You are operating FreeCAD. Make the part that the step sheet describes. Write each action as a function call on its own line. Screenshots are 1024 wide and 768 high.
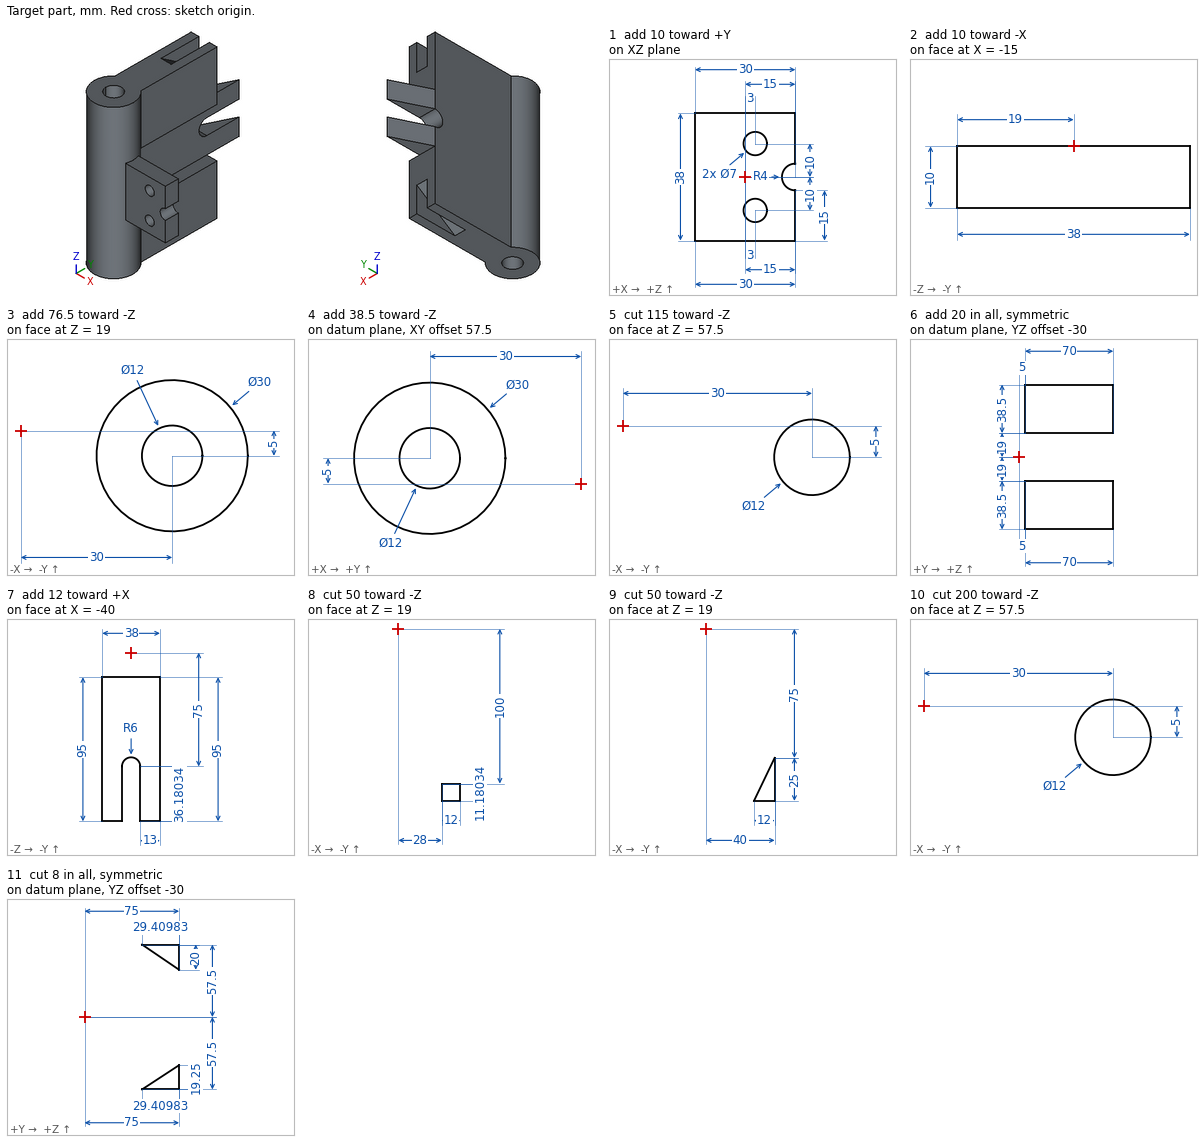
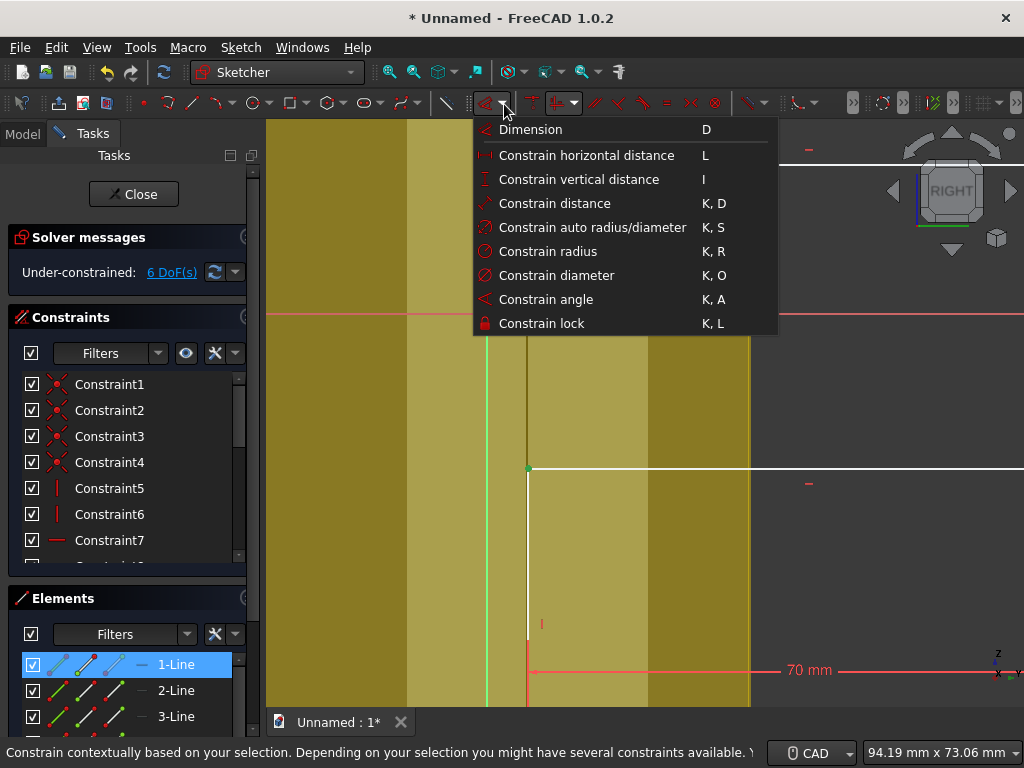
click(626, 155)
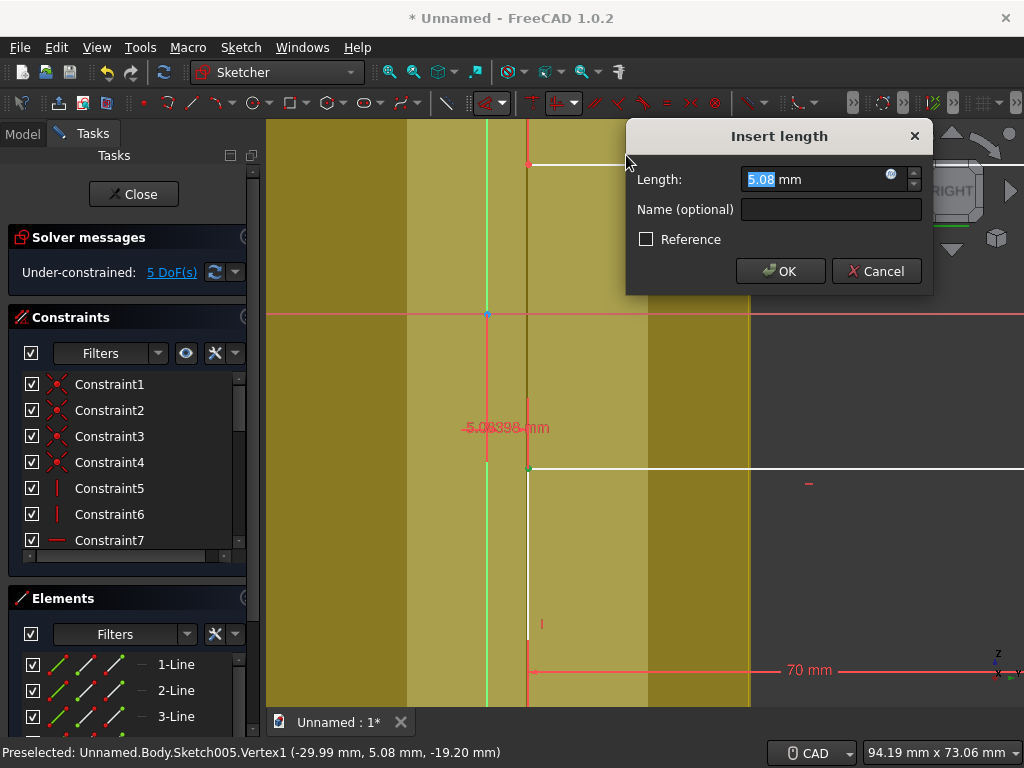
text(5)
key(Return)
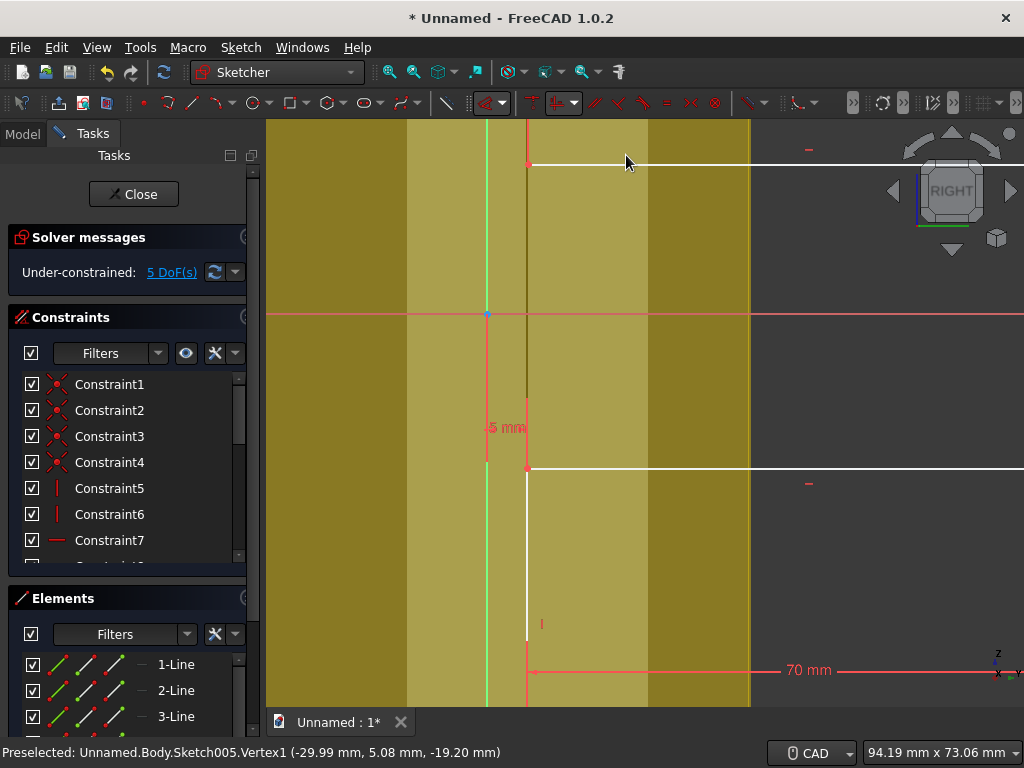
scroll(453, 470, down, 5)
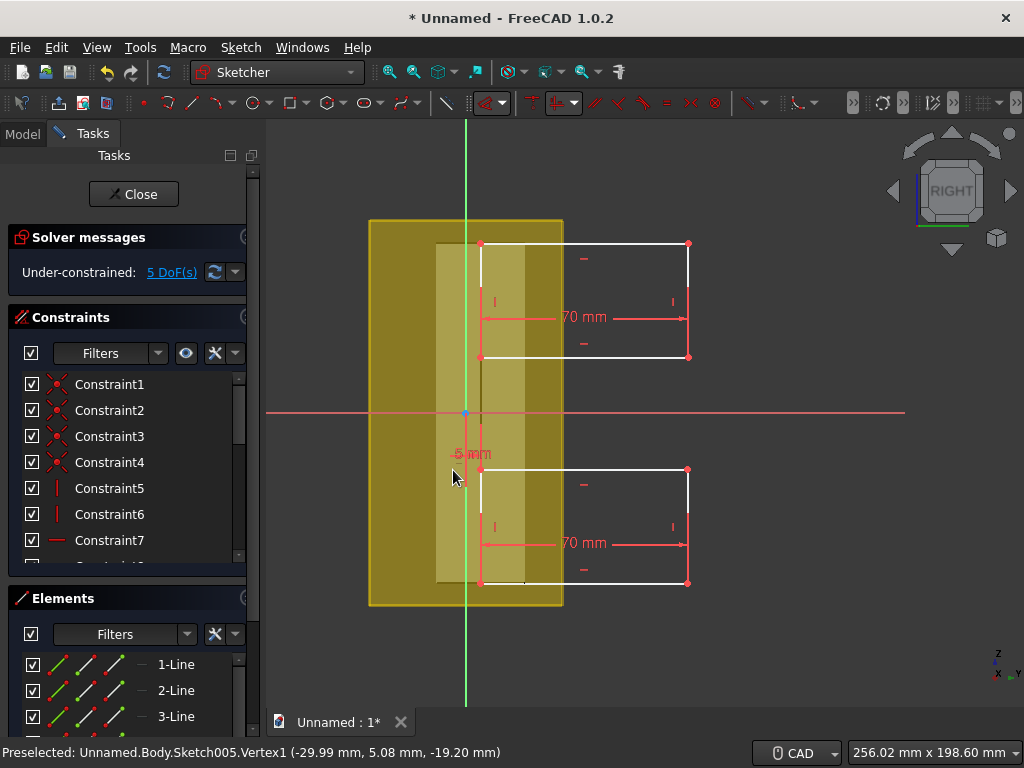
scroll(481, 244, up, 5)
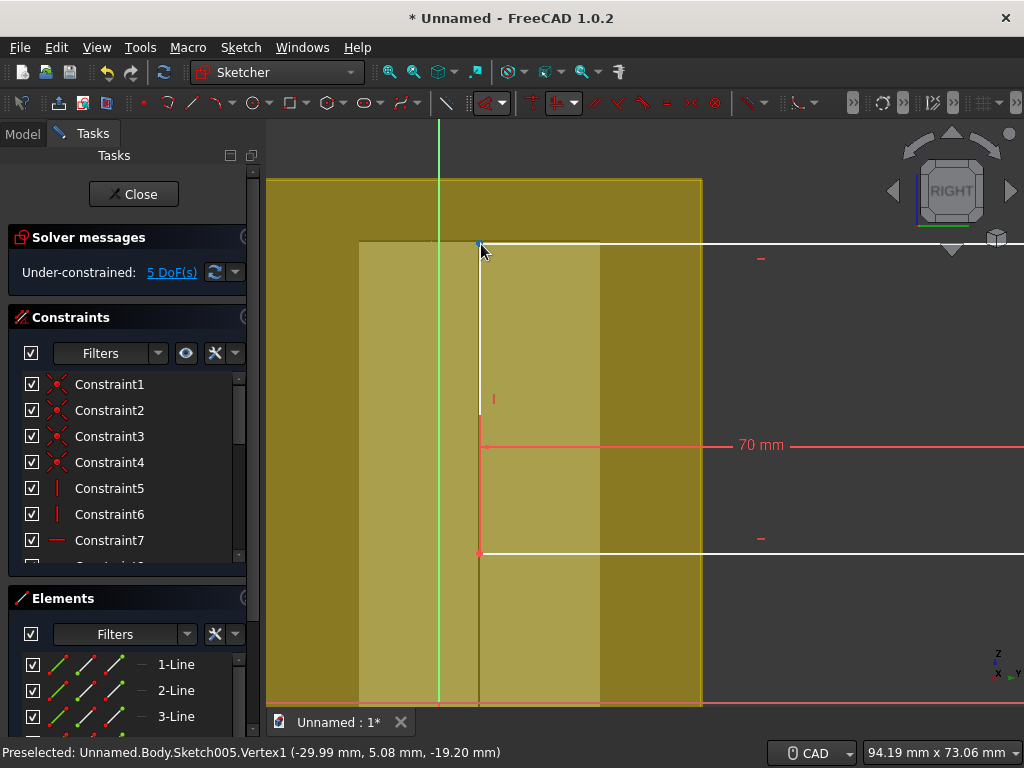
click(480, 244)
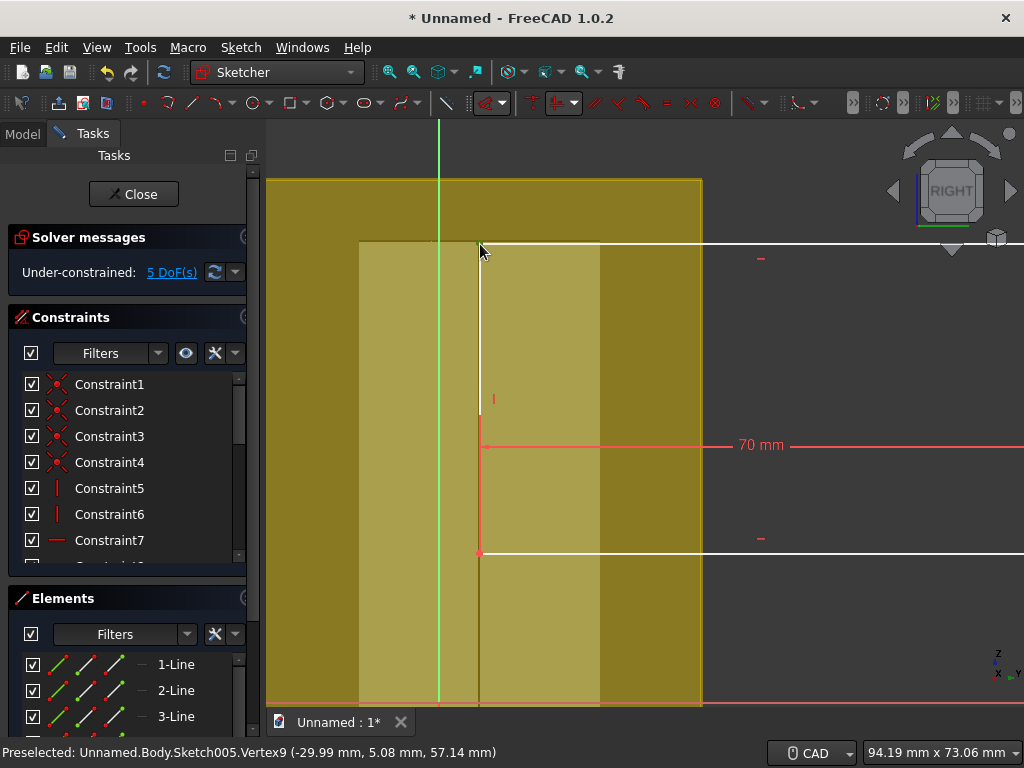
click(504, 104)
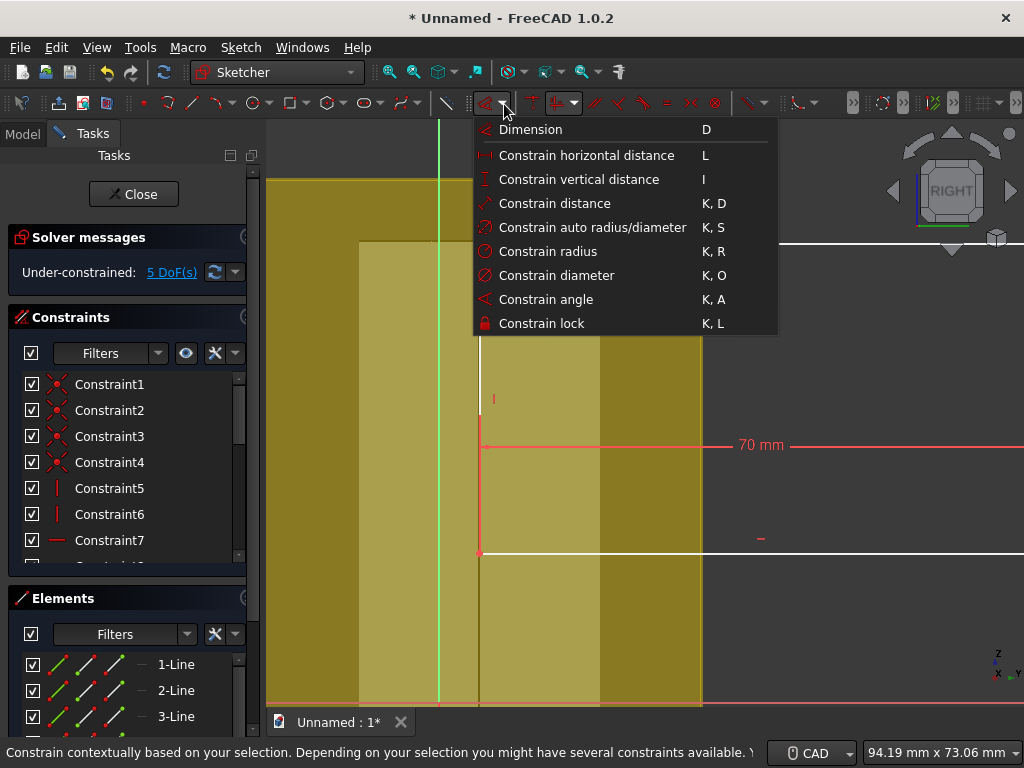
click(626, 155)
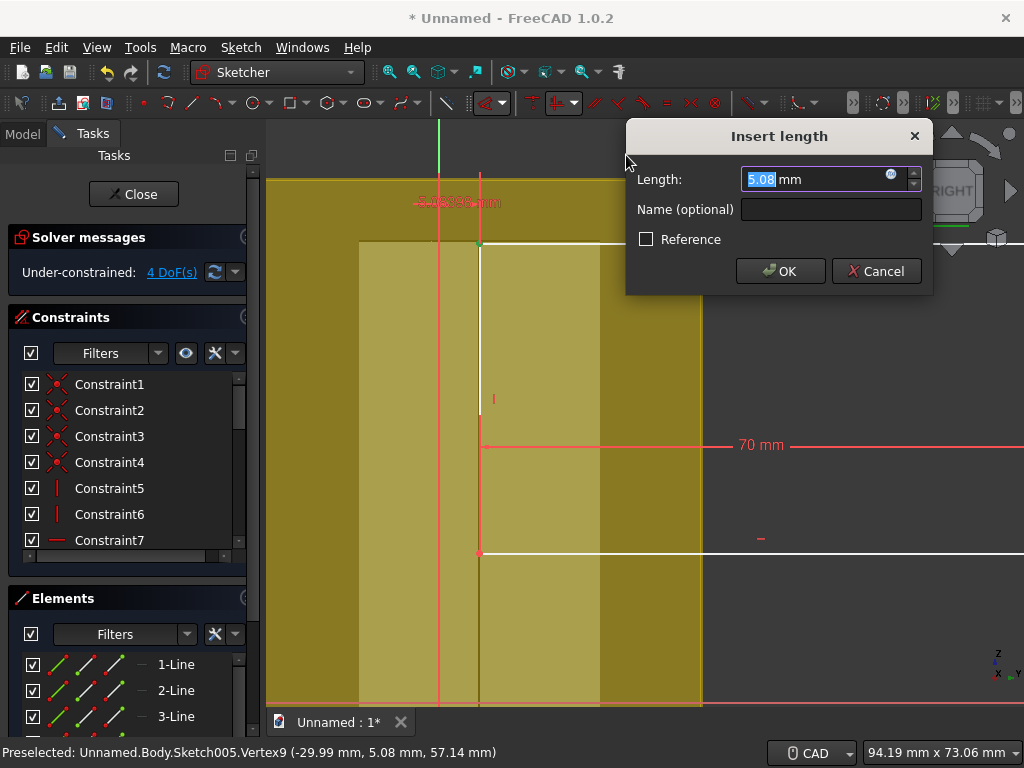
text(5)
key(Return)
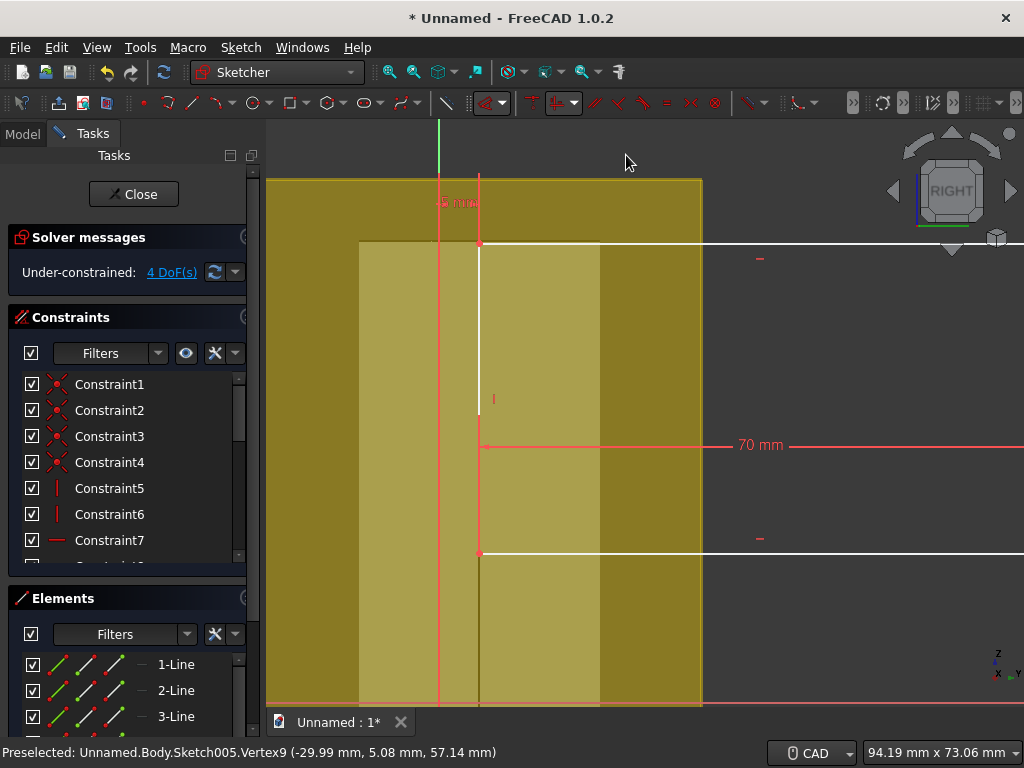
scroll(481, 244, down, 5)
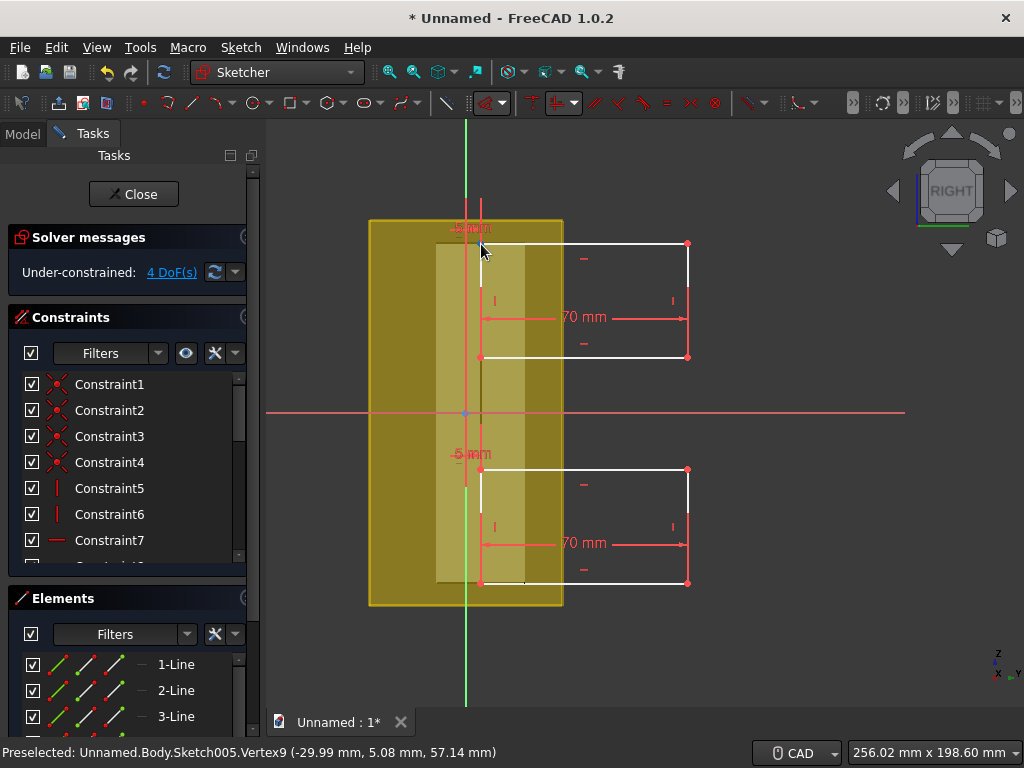
click(481, 470)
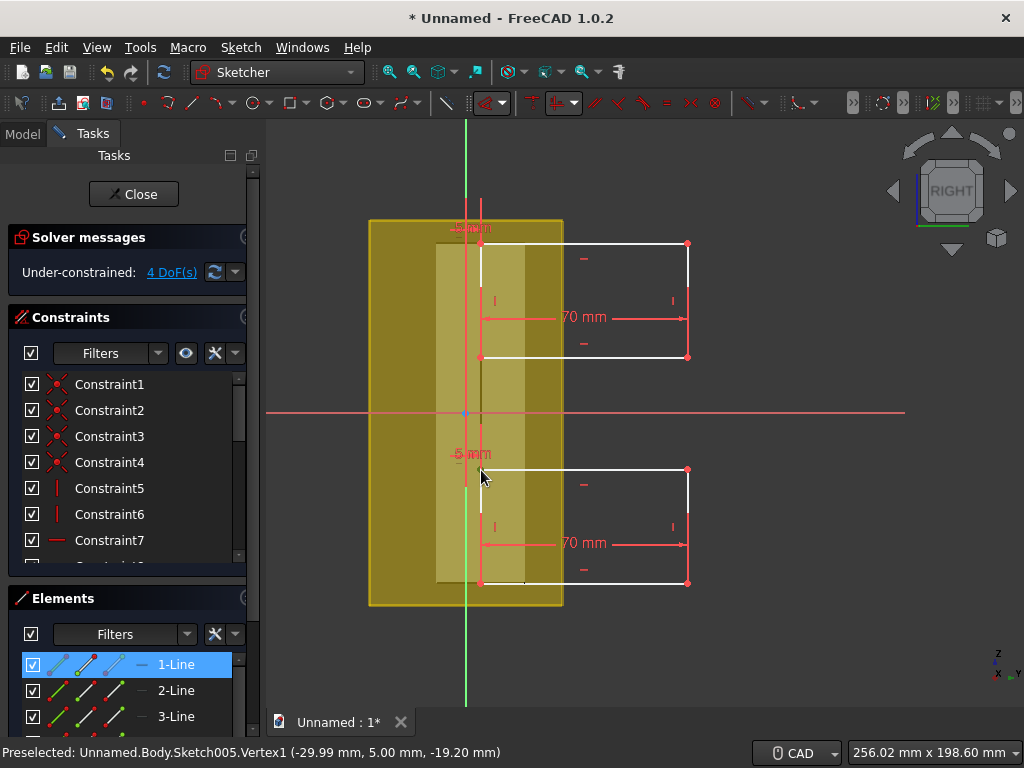
key(i)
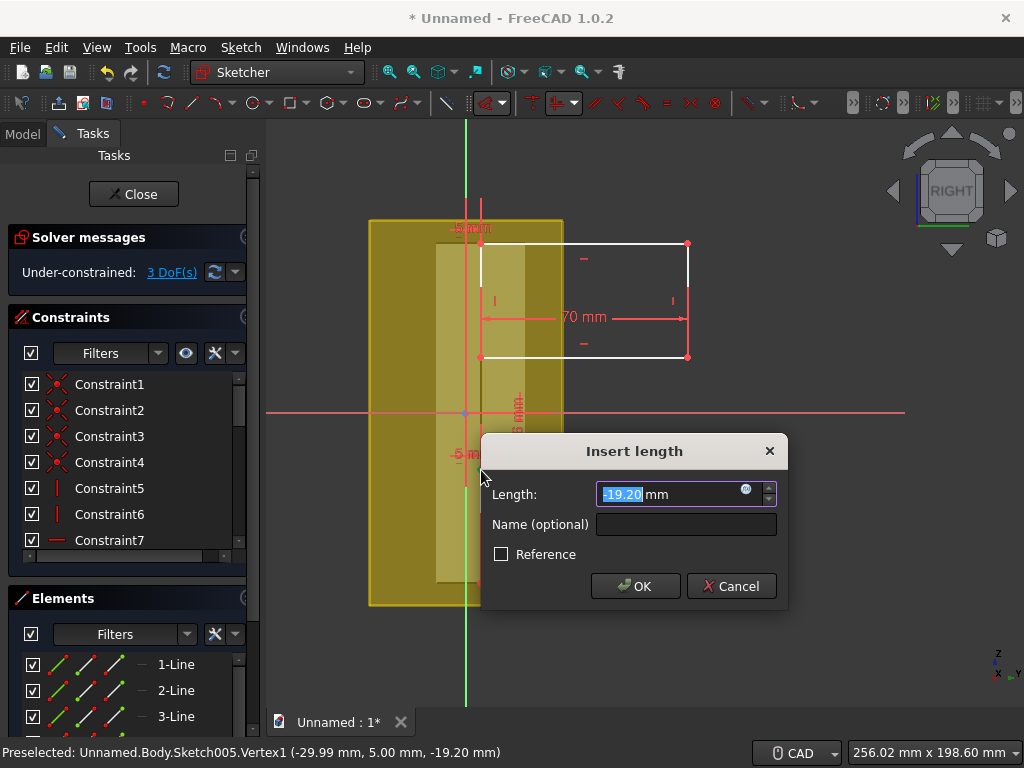
text(-19)
key(Return)